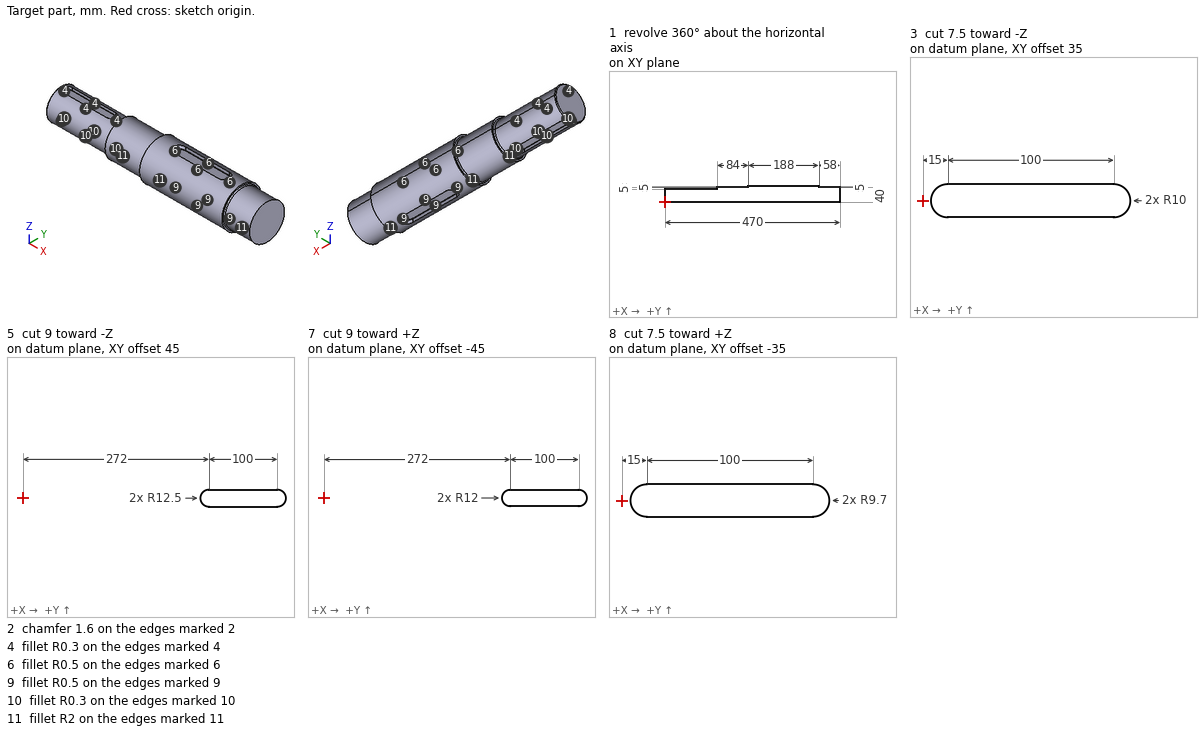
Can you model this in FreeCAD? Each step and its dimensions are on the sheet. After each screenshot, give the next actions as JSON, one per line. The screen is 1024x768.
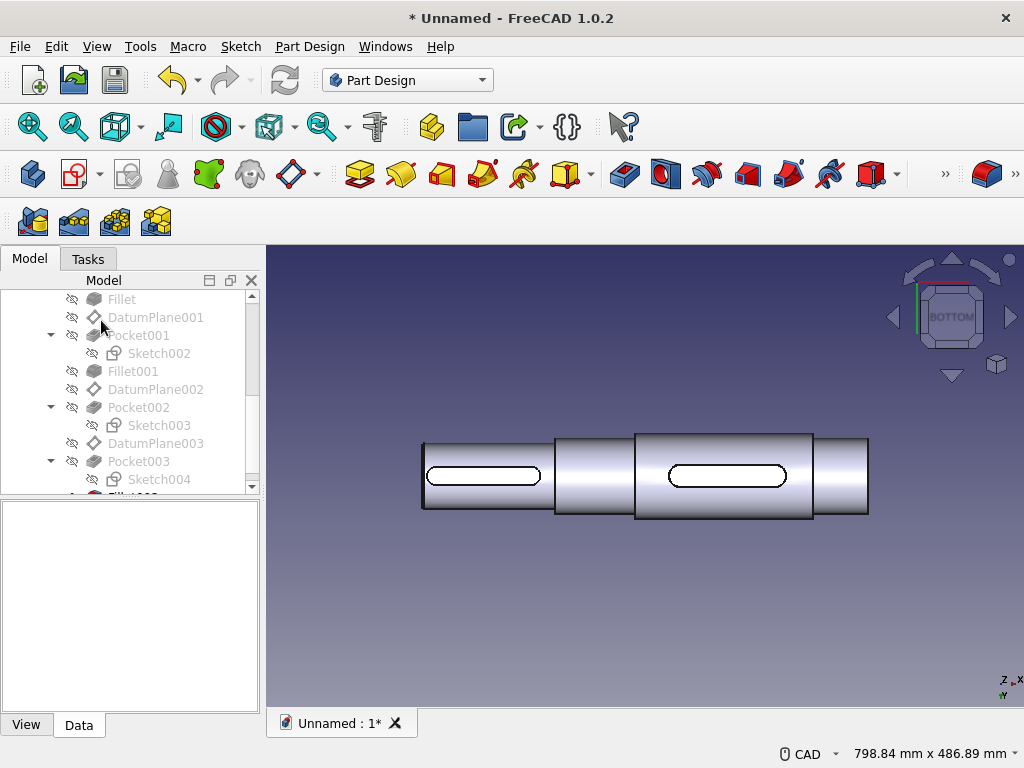
{"action": "left_click", "coordinate": [516, 475]}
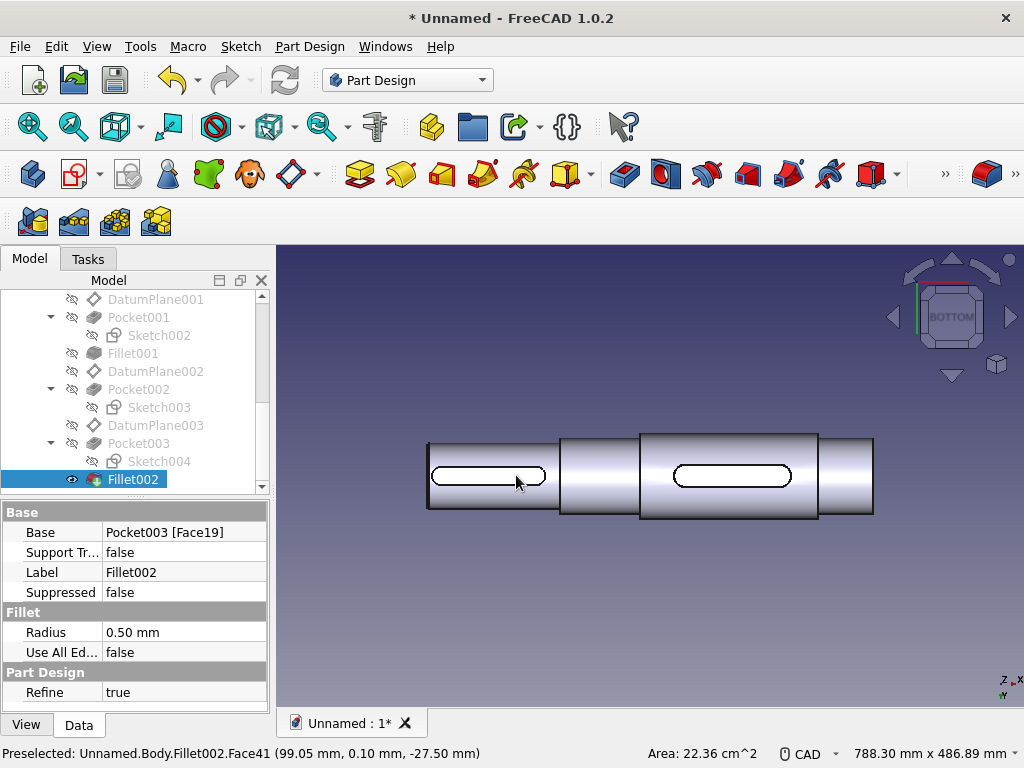
{"action": "left_click", "coordinate": [987, 174]}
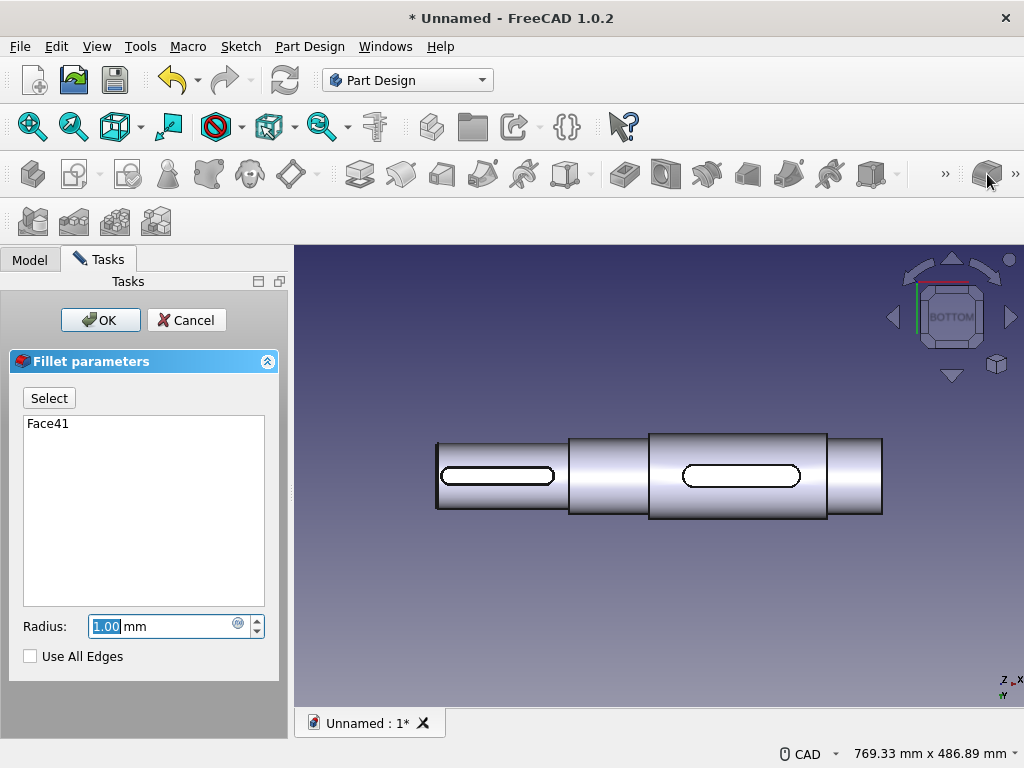
{"action": "type", "text": "0.3"}
{"action": "key", "text": "Tab"}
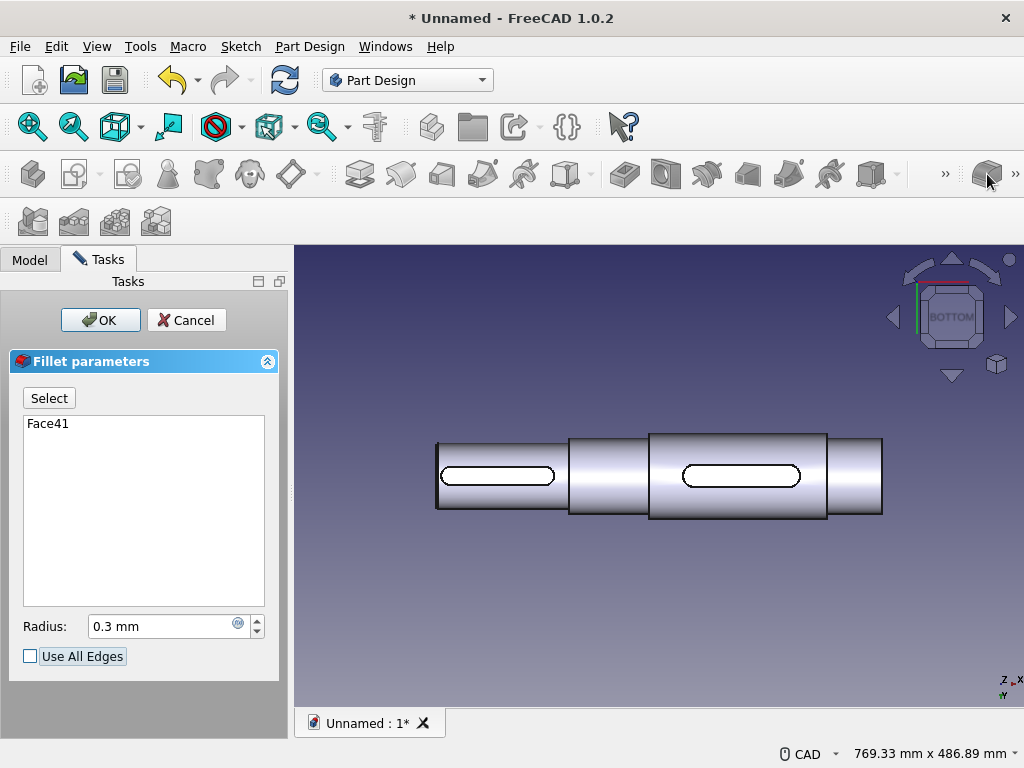
{"action": "left_click", "coordinate": [101, 320]}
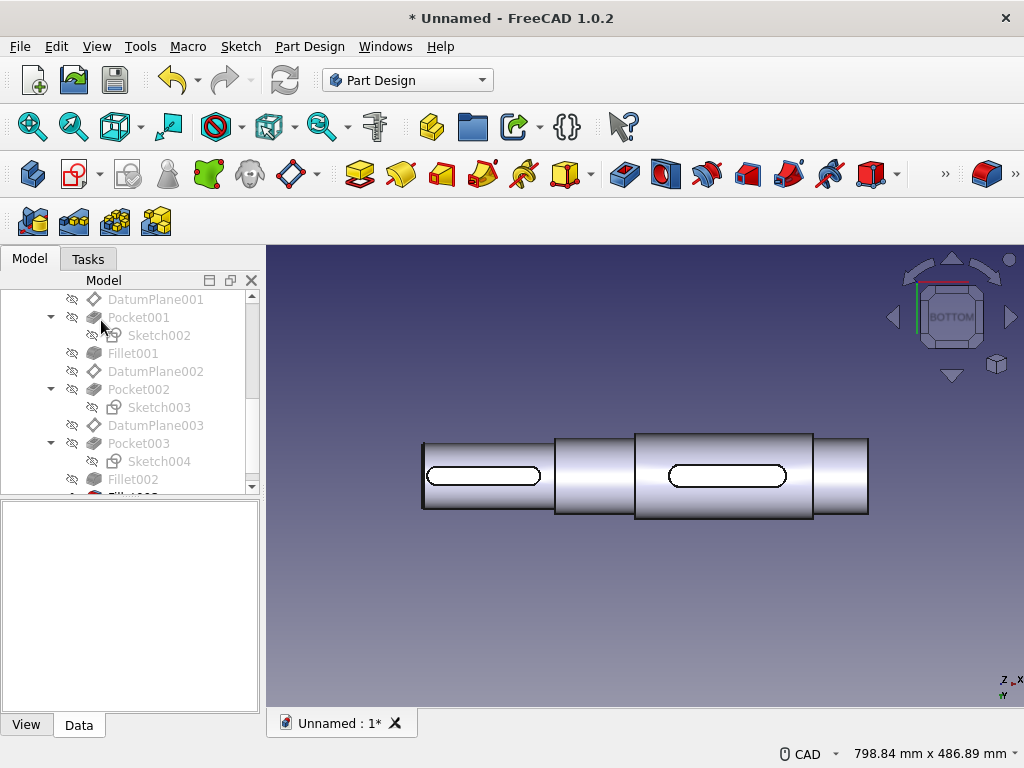
{"action": "key", "text": "0"}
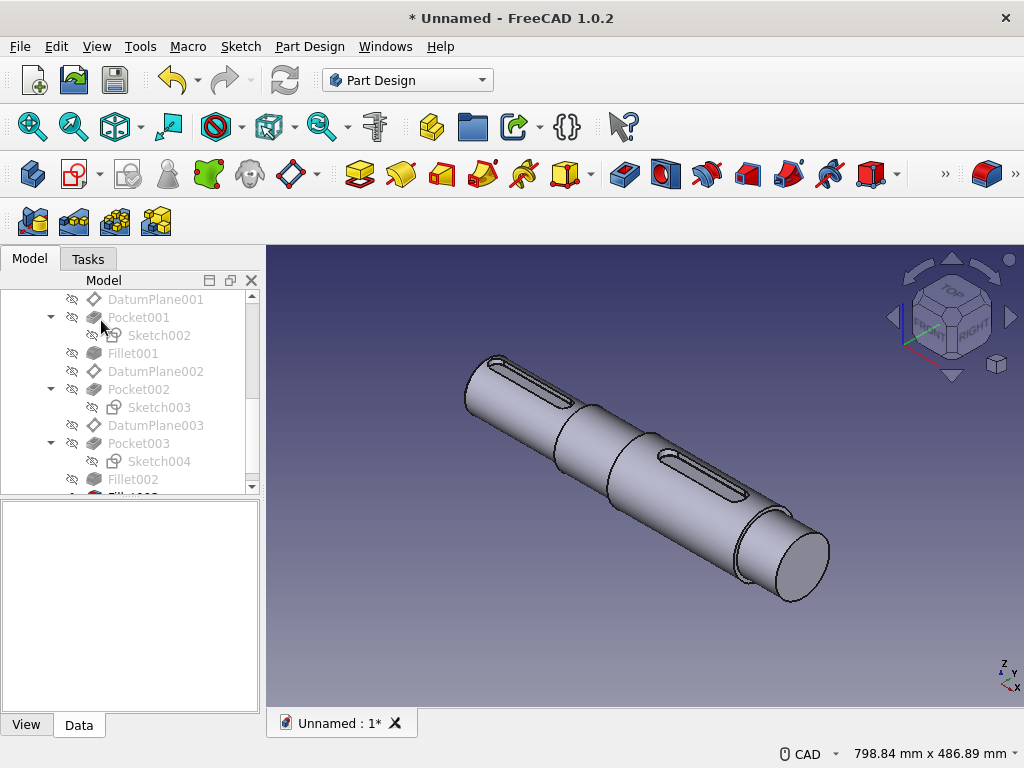
{"action": "key", "text": "2"}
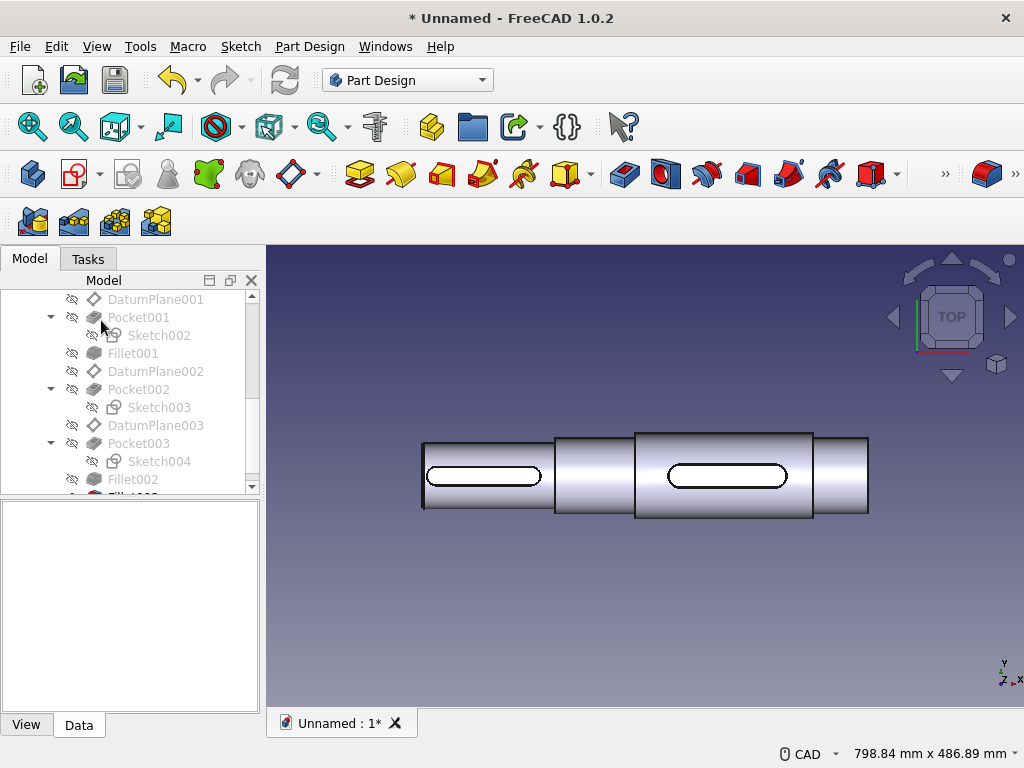
{"action": "key", "text": "1"}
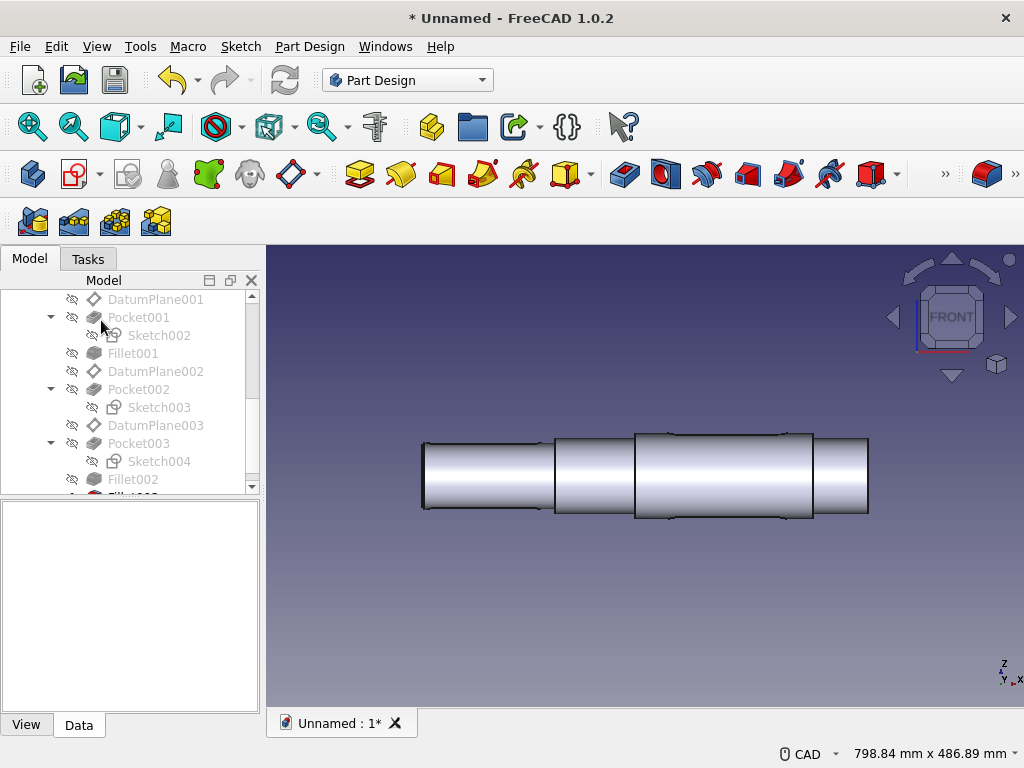
{"action": "key", "text": "3"}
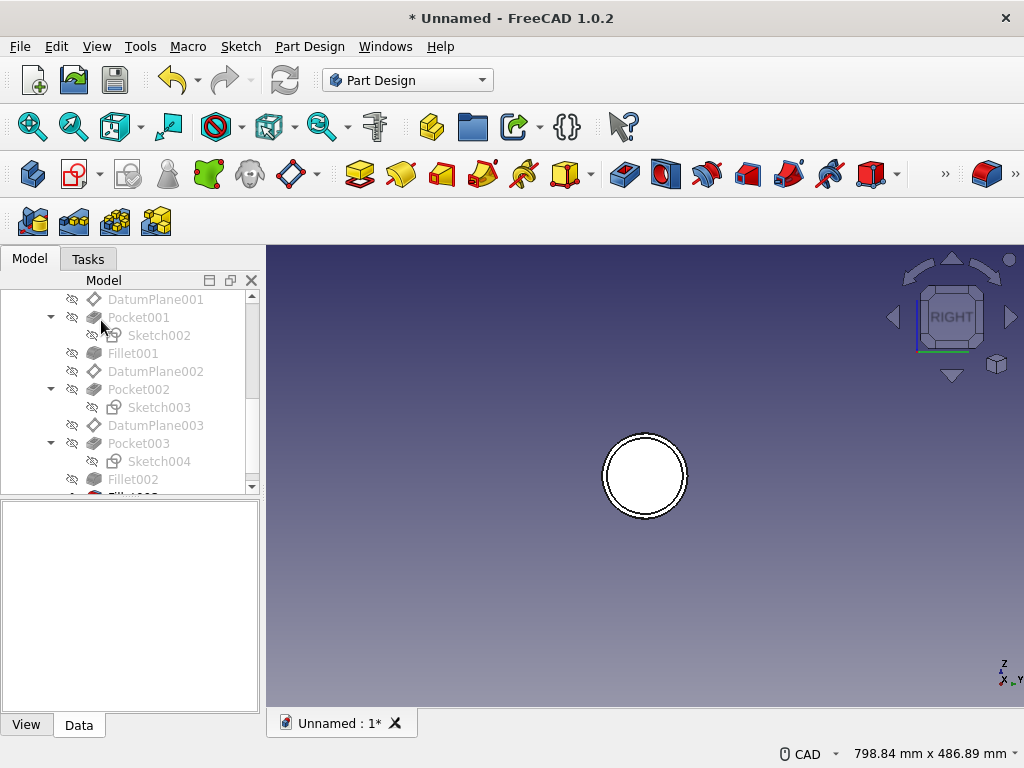
{"action": "left_click", "coordinate": [33, 128]}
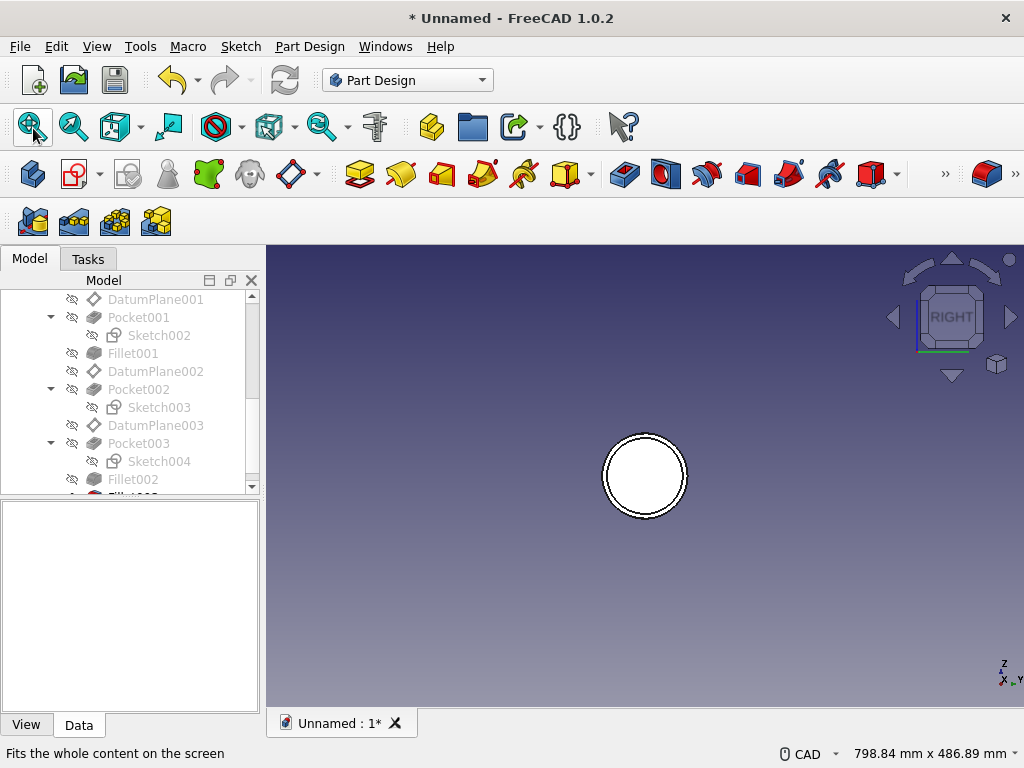
{"action": "key", "text": "5"}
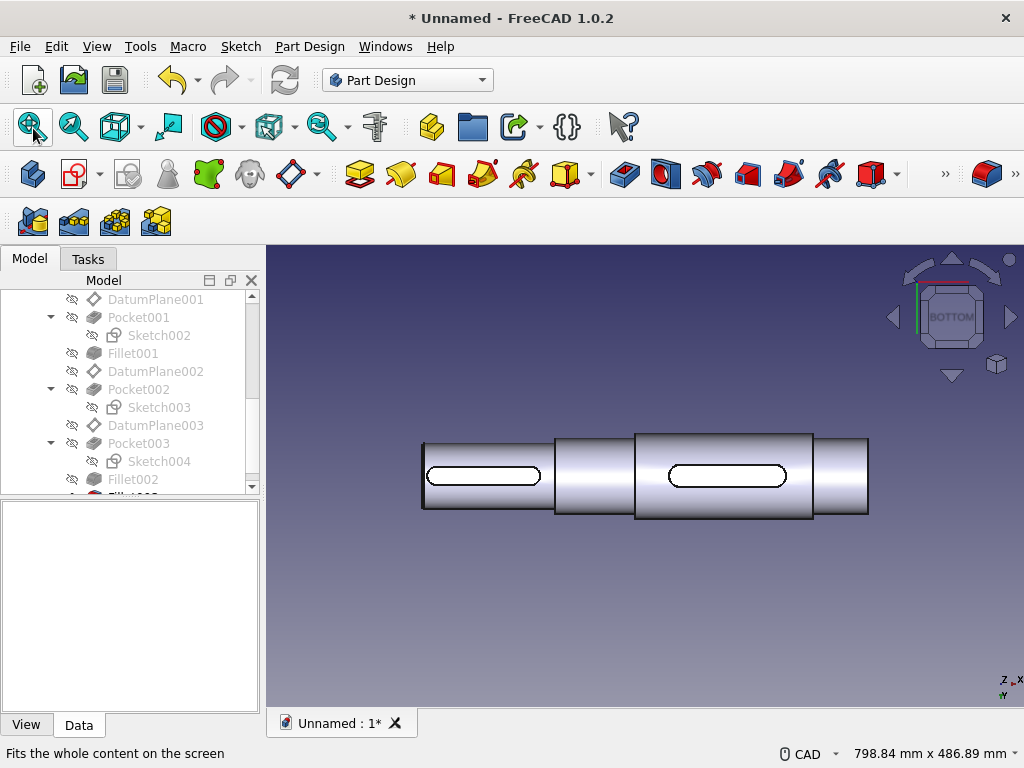
{"action": "key", "text": "4"}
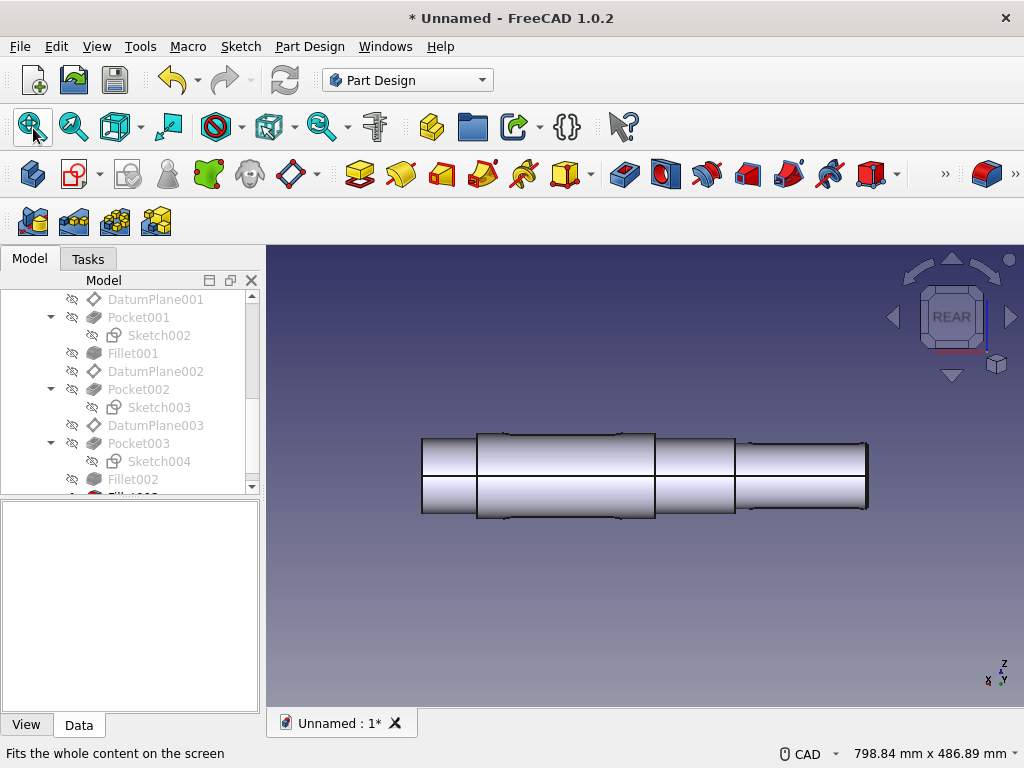
{"action": "key", "text": "6"}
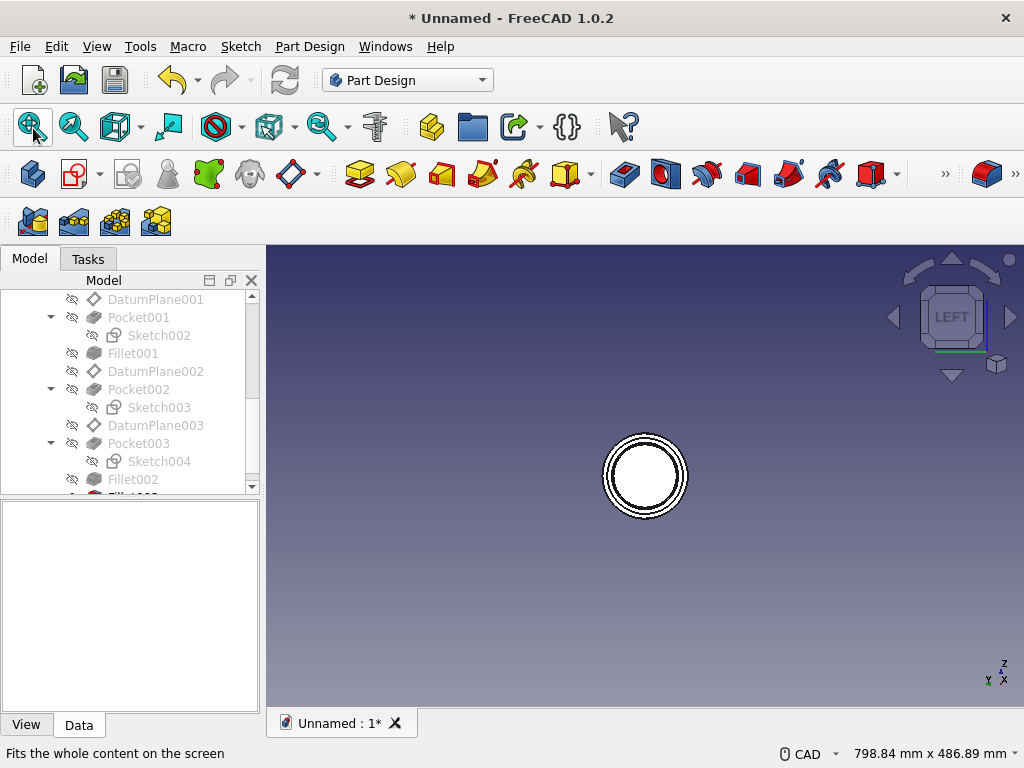
{"action": "left_click", "coordinate": [33, 128]}